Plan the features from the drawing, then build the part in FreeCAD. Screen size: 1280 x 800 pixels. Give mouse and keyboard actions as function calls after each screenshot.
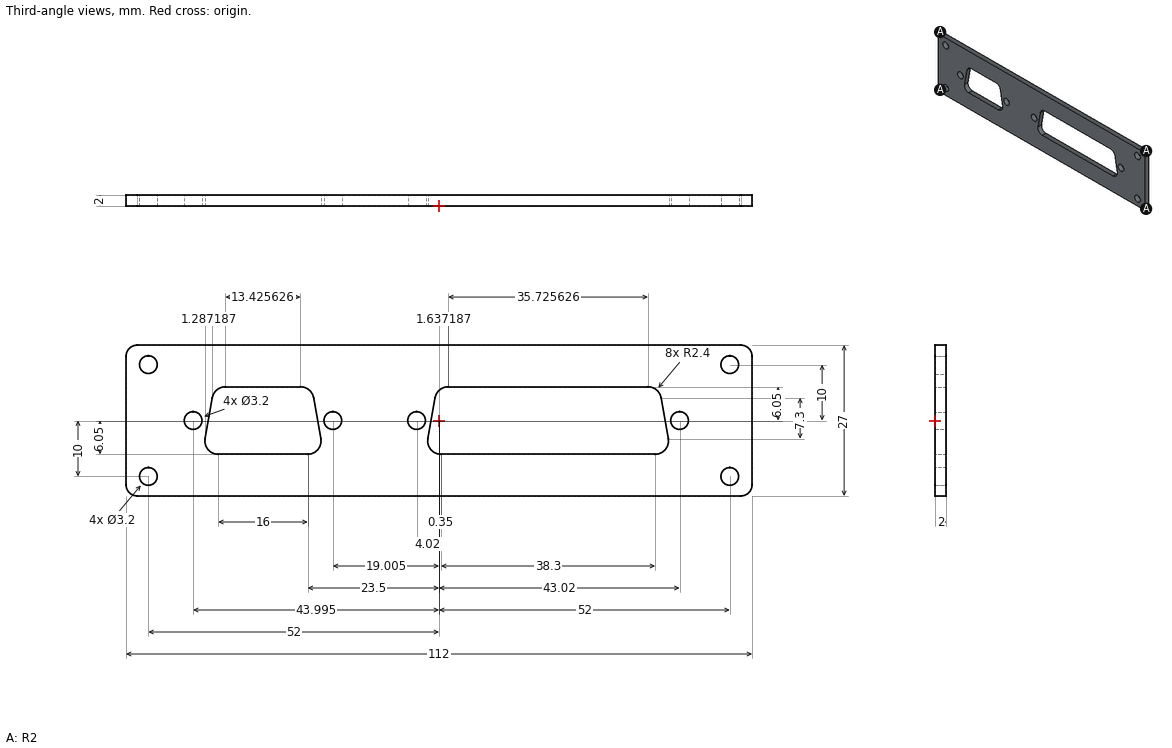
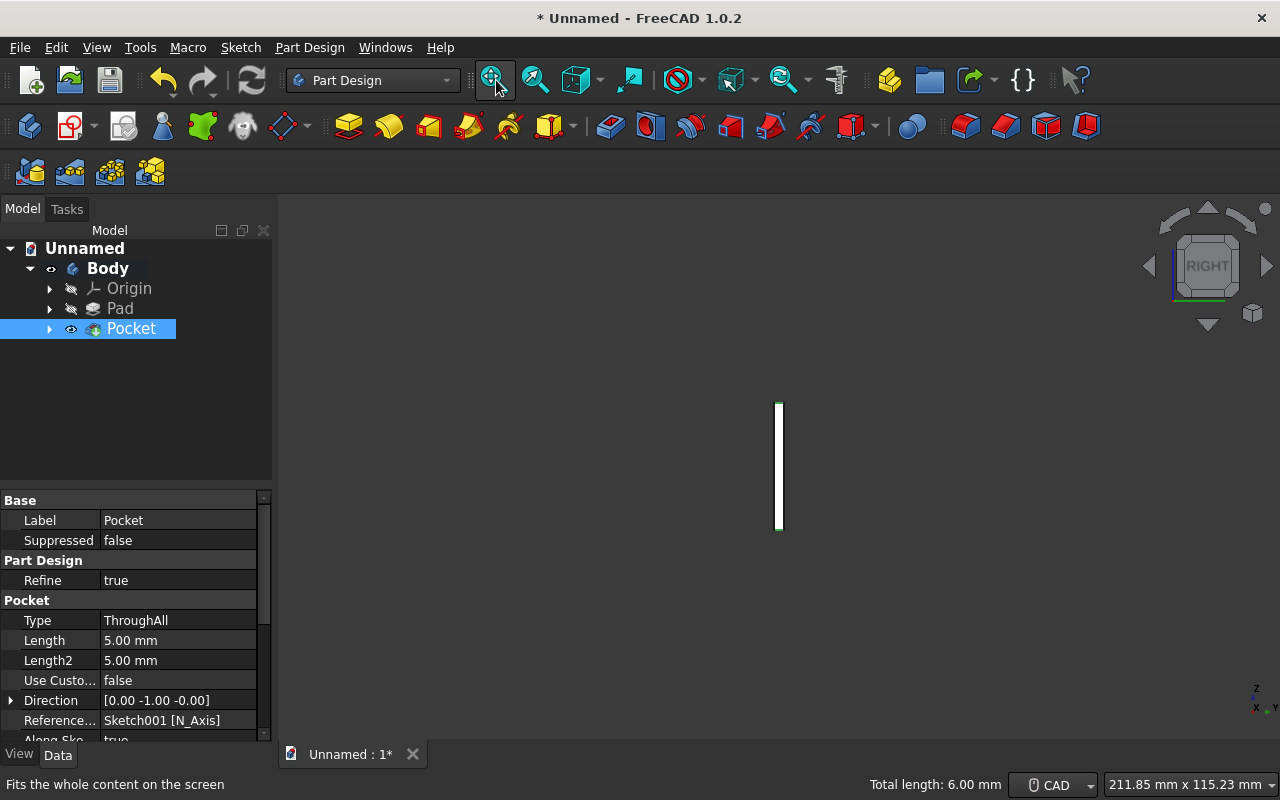
key(5)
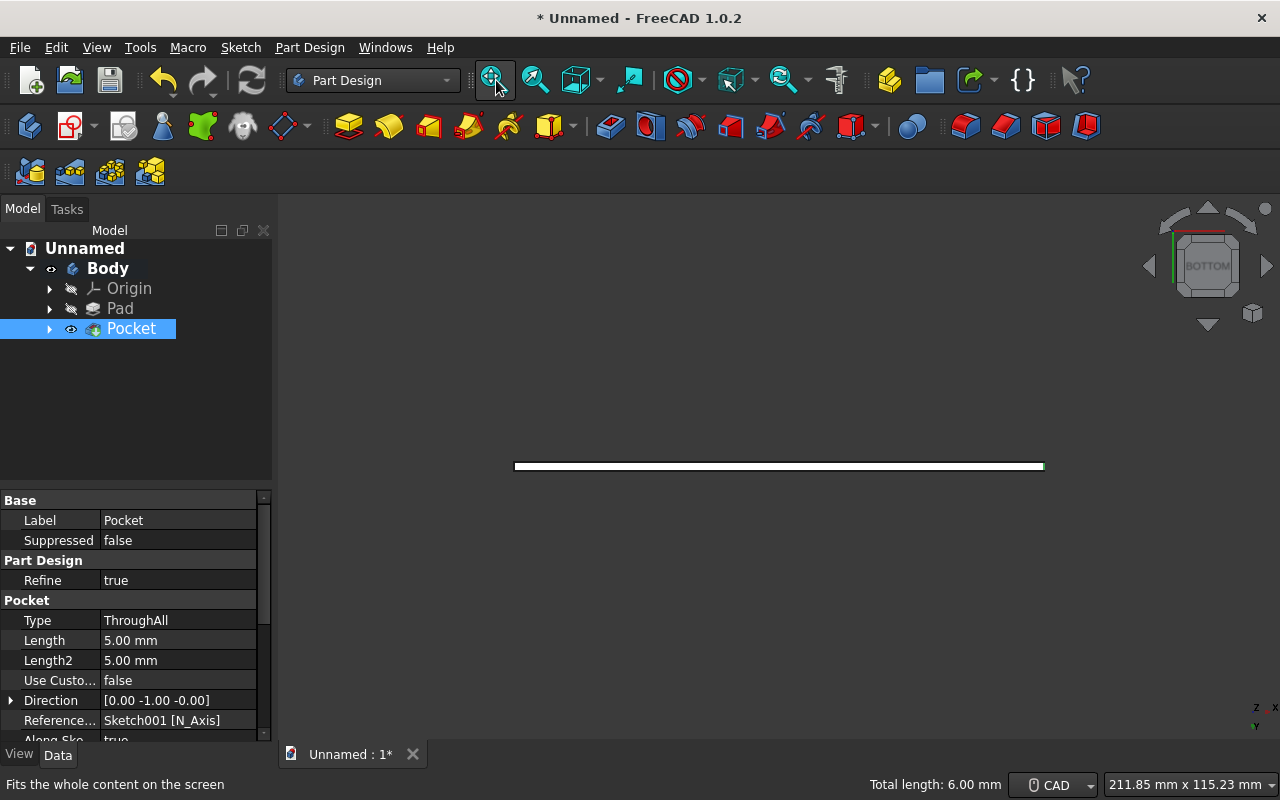
click(514, 467, ctrl)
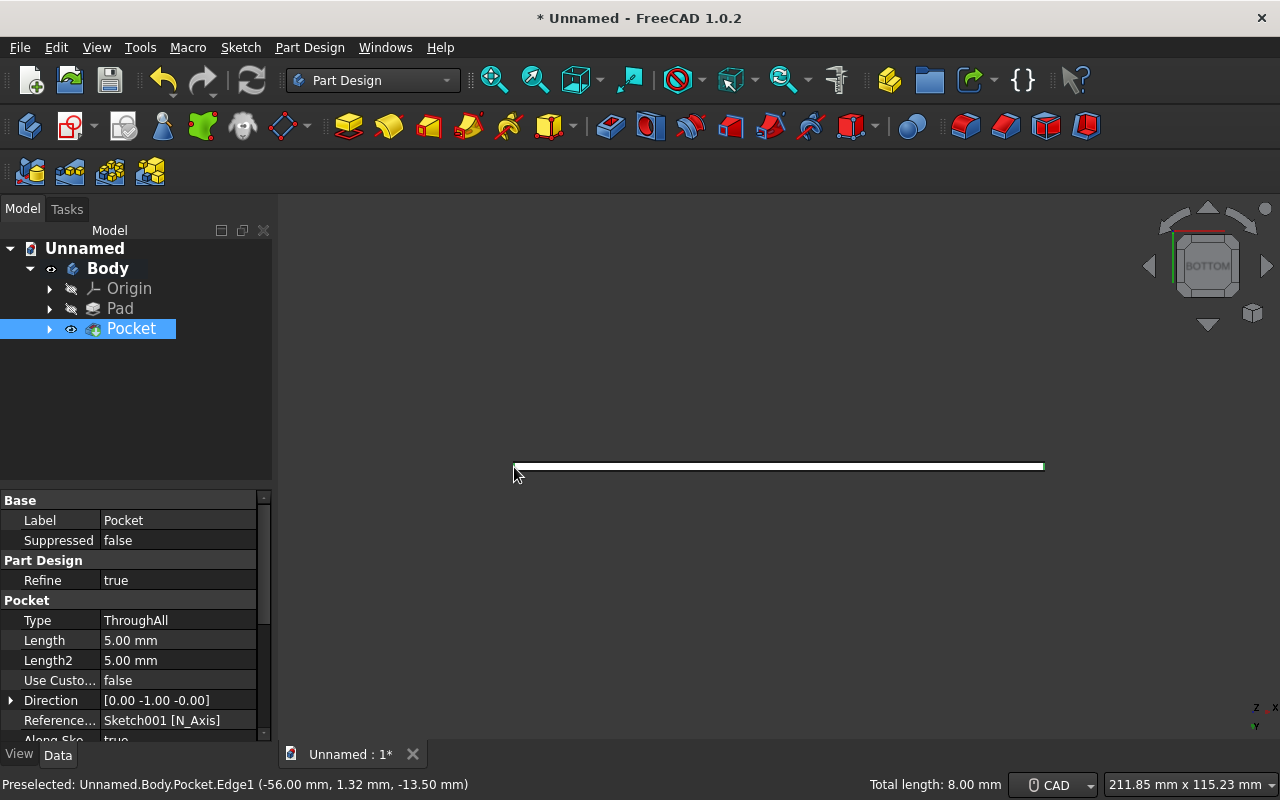
click(966, 126)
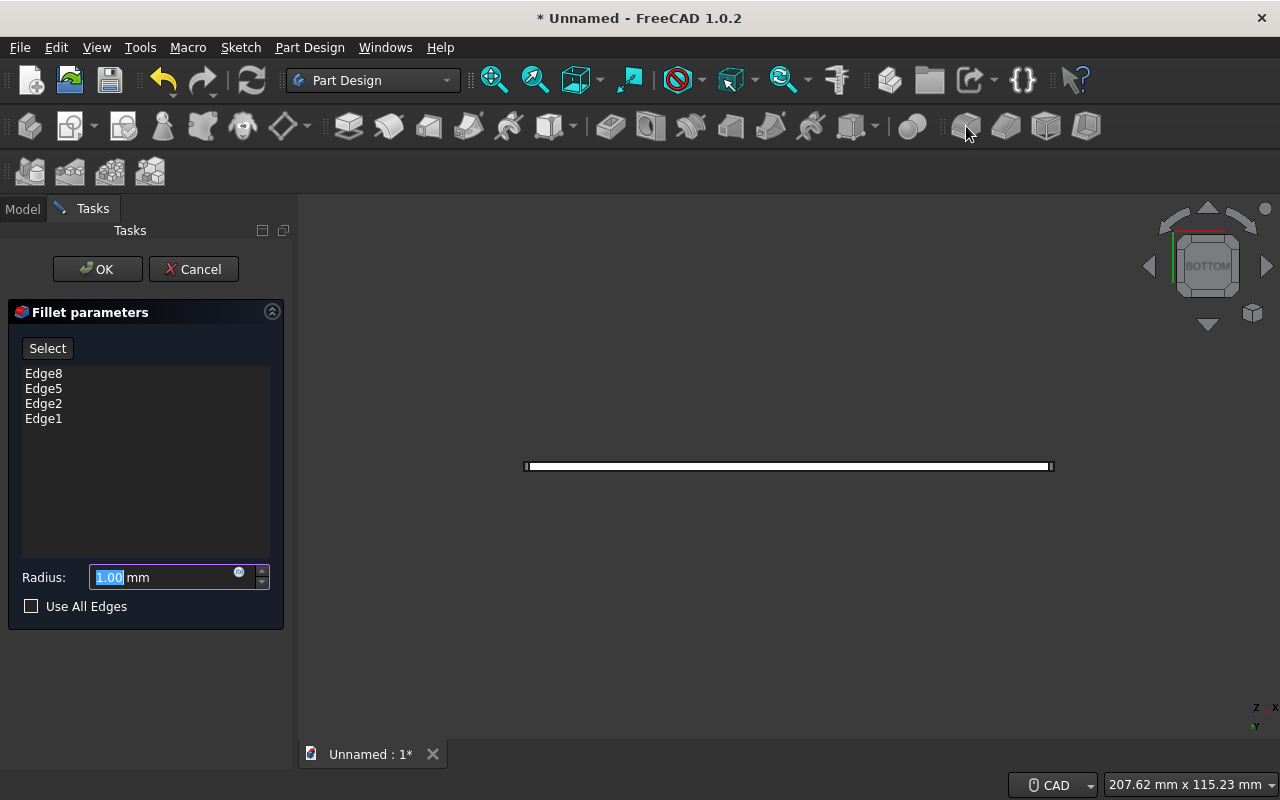
text(2)
key(Tab)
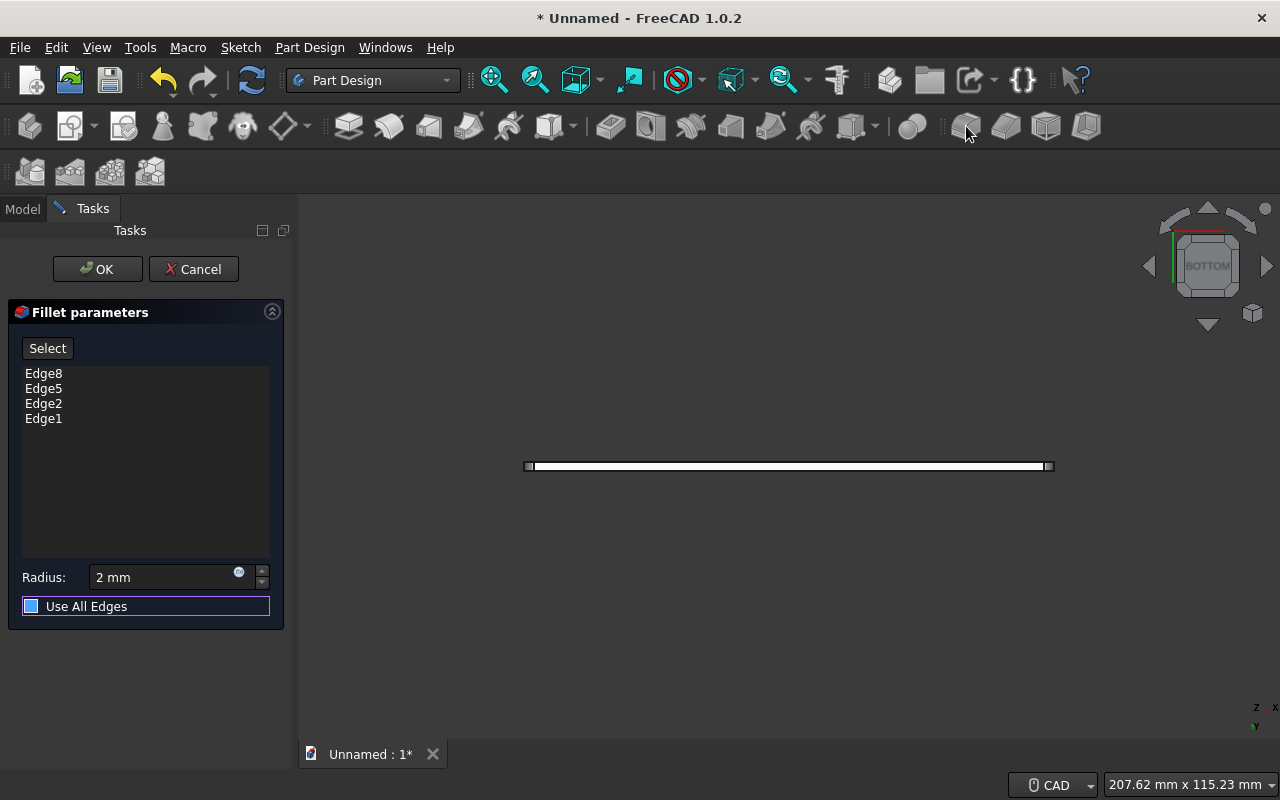
click(98, 269)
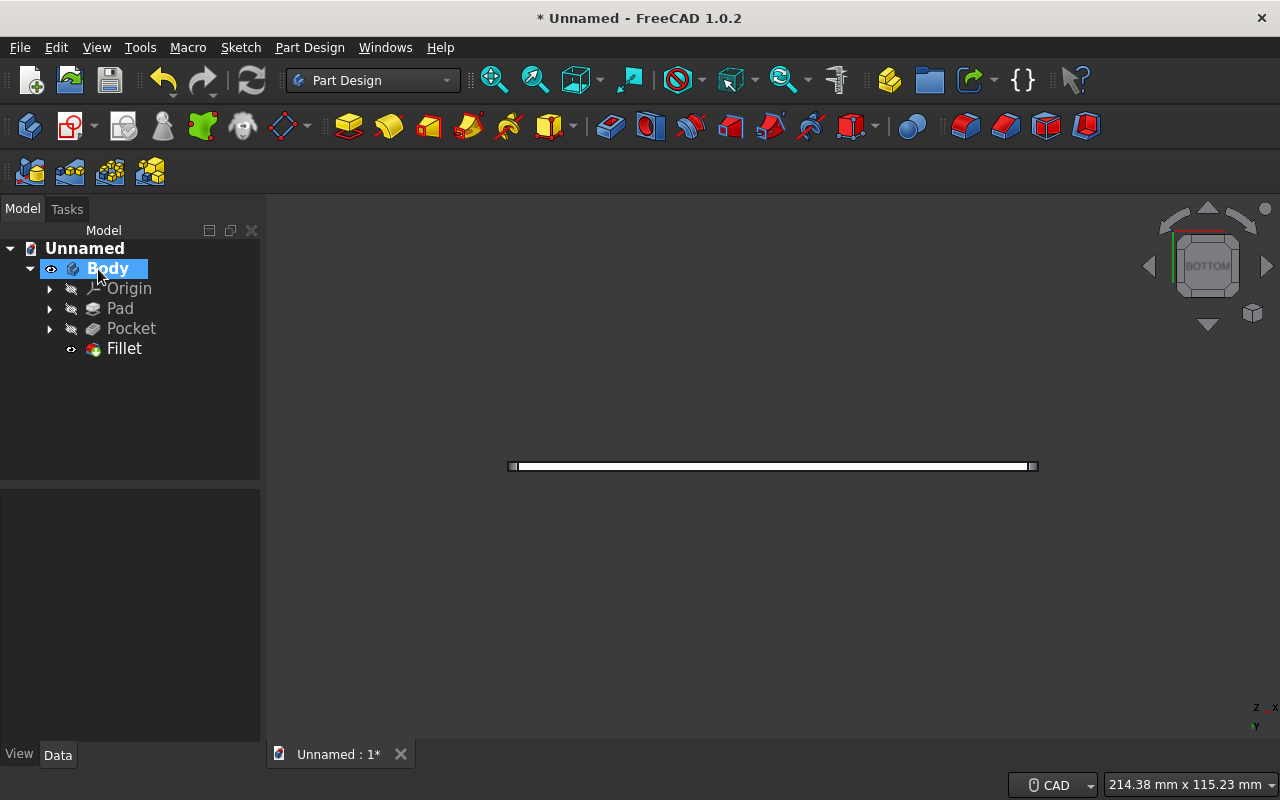
key(4)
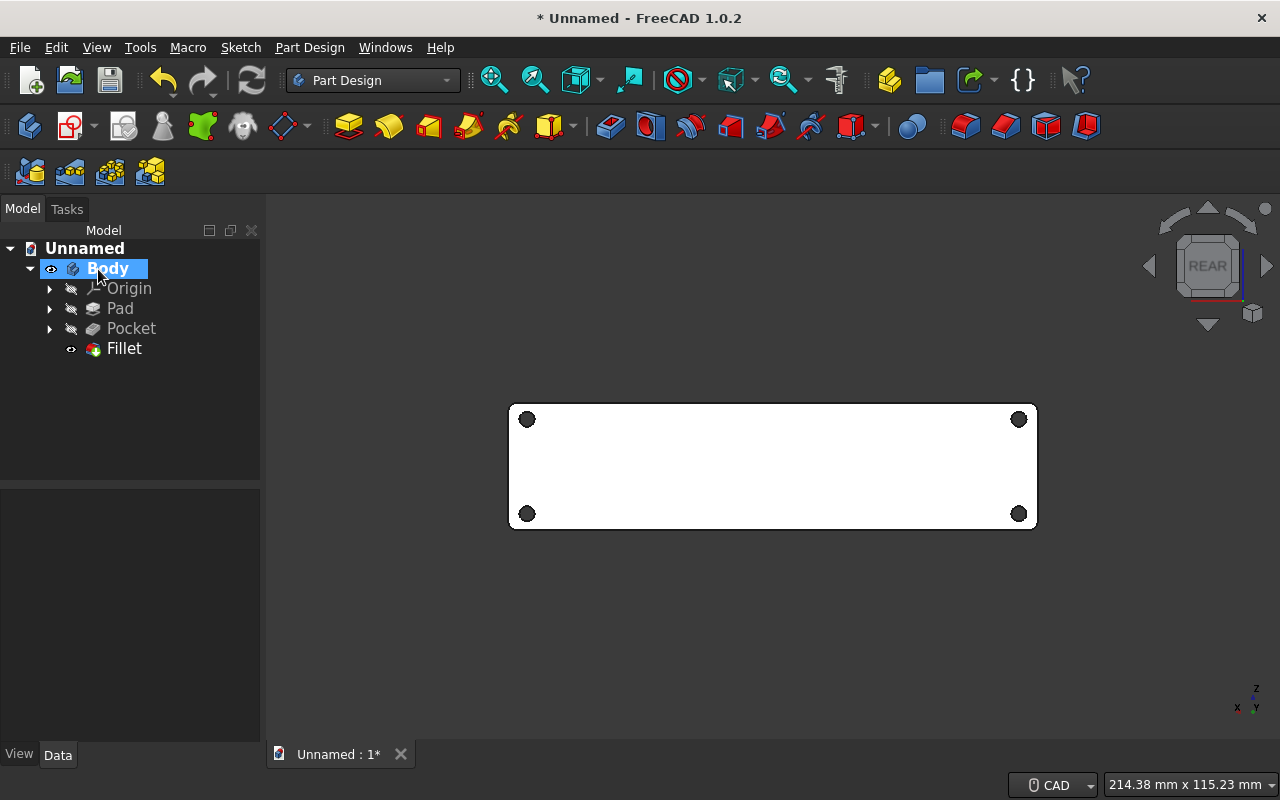
click(622, 466)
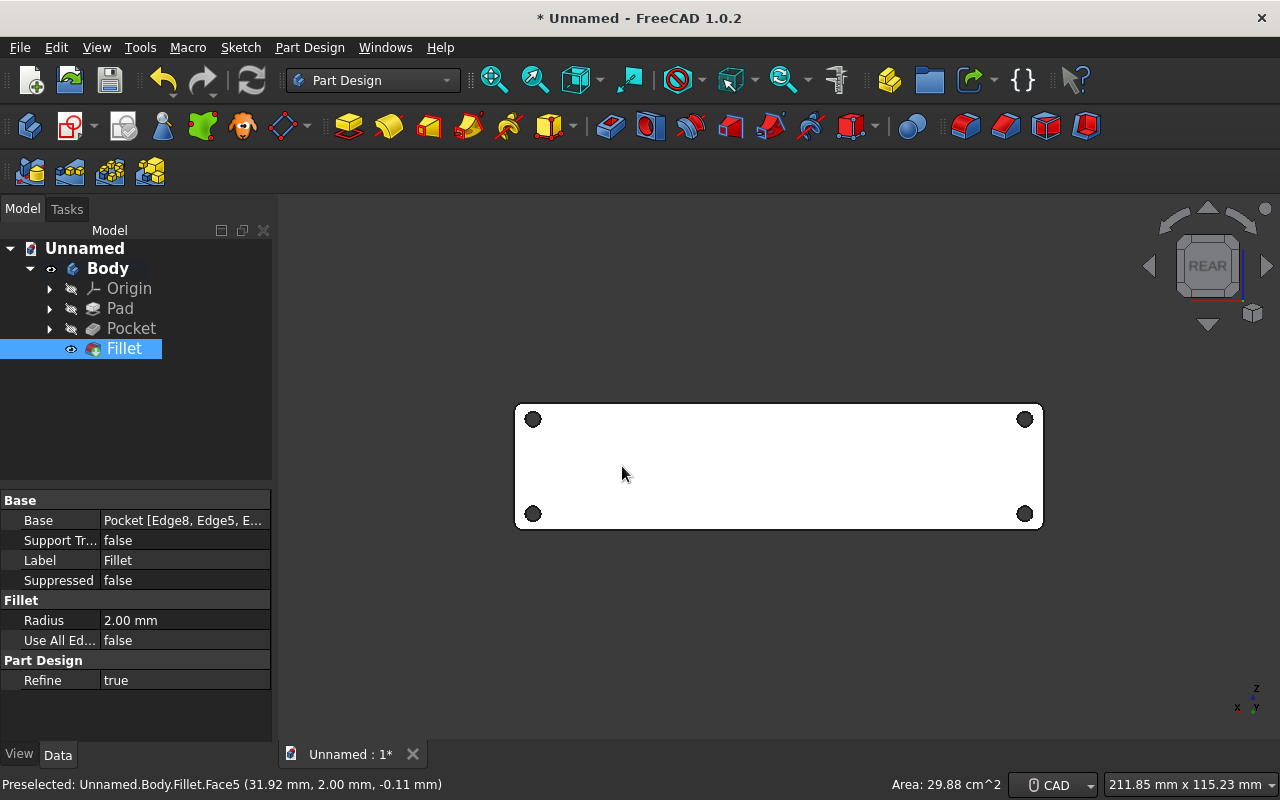
click(70, 126)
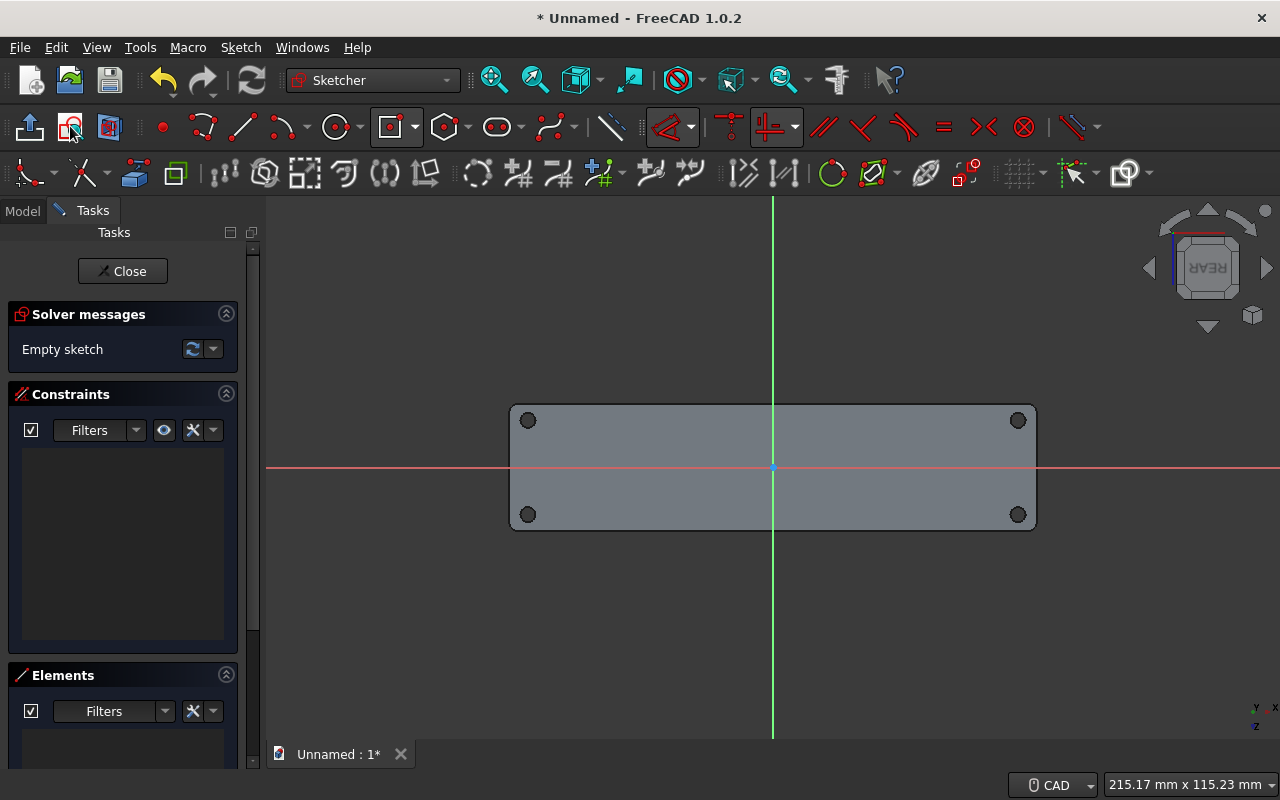
scroll(905, 467, up, 2)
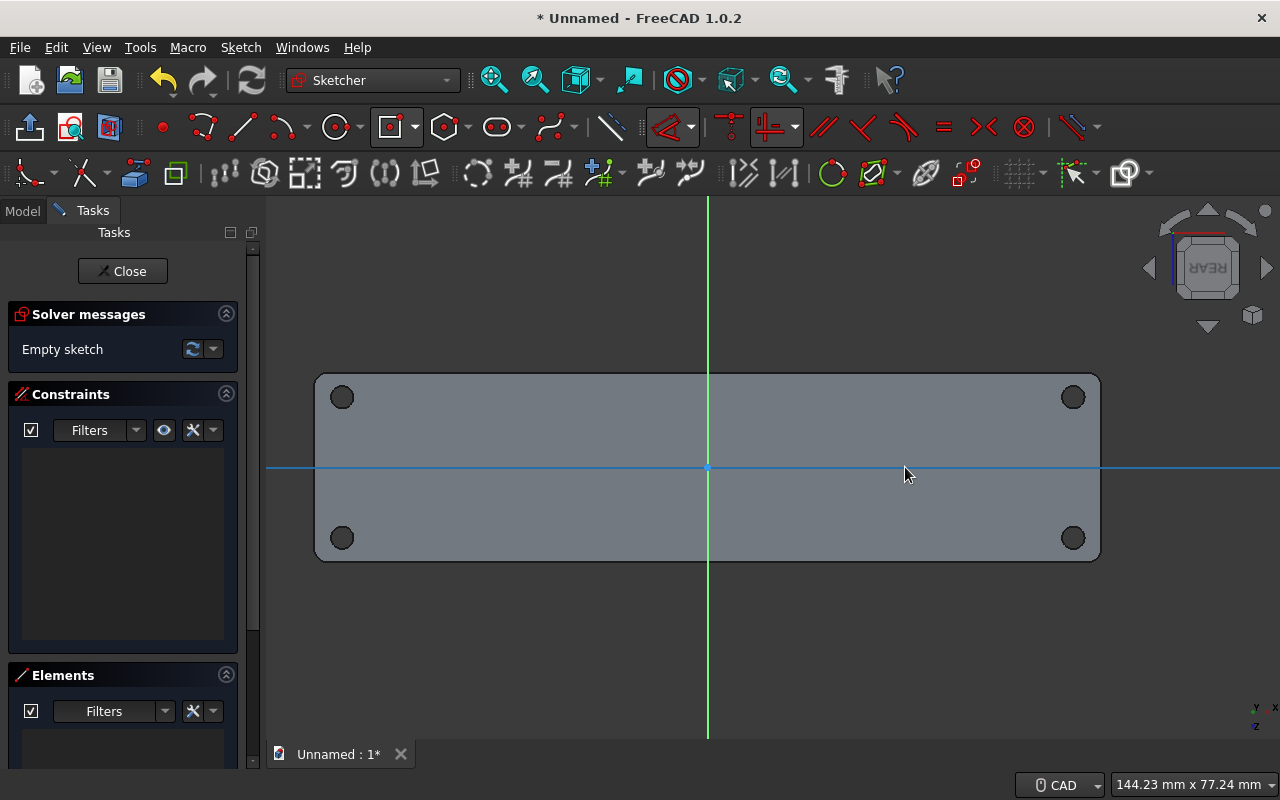
click(244, 128)